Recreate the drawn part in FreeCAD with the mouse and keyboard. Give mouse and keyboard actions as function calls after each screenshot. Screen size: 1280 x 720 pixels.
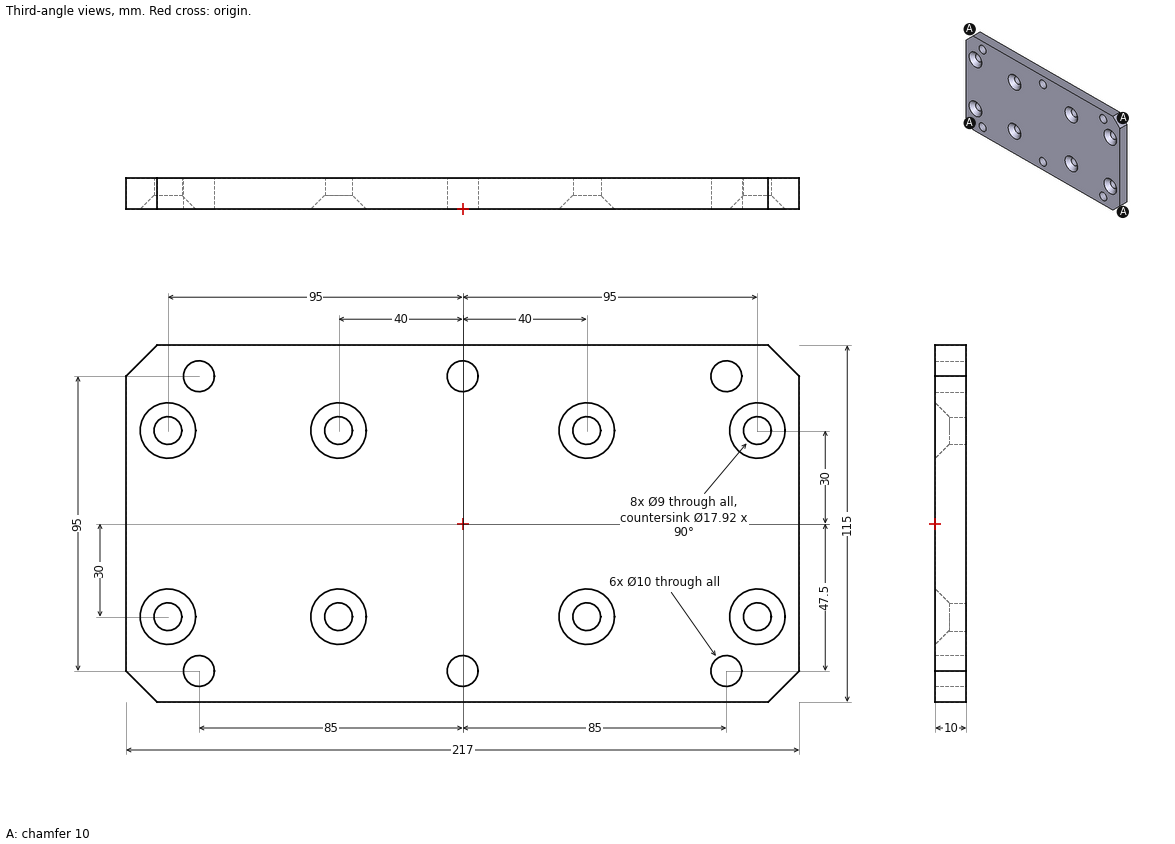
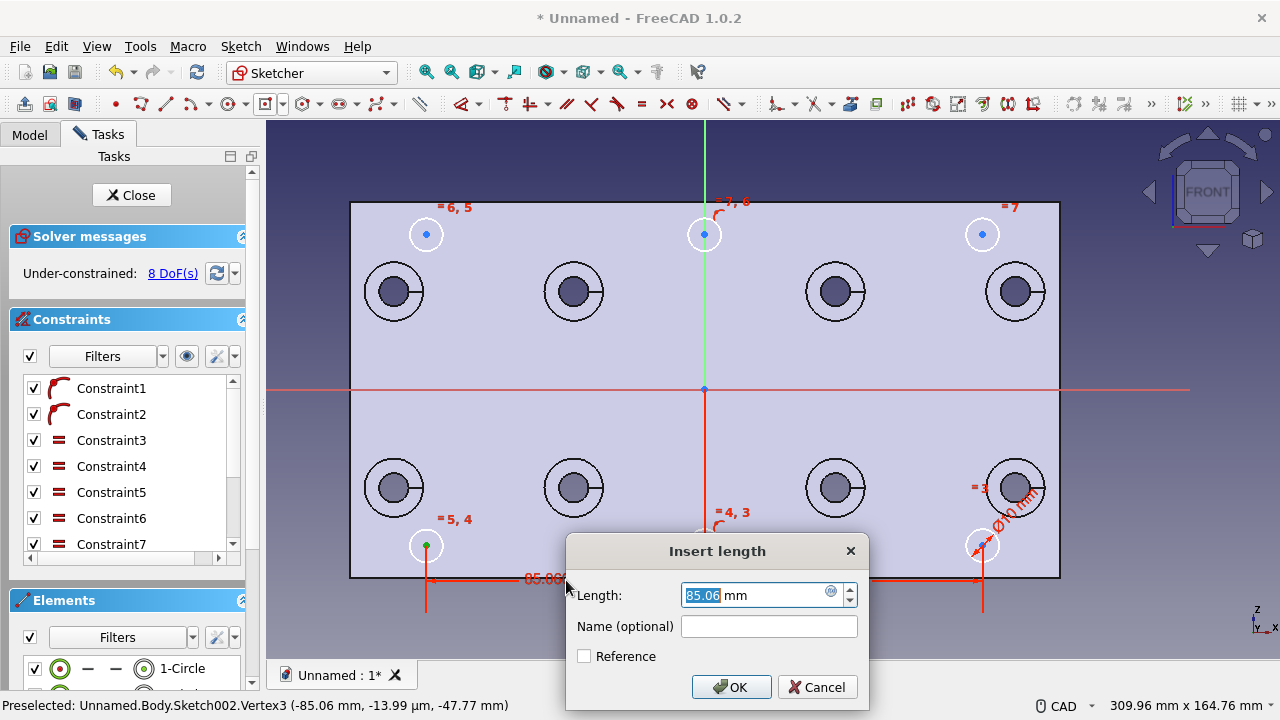
text(85)
key(Return)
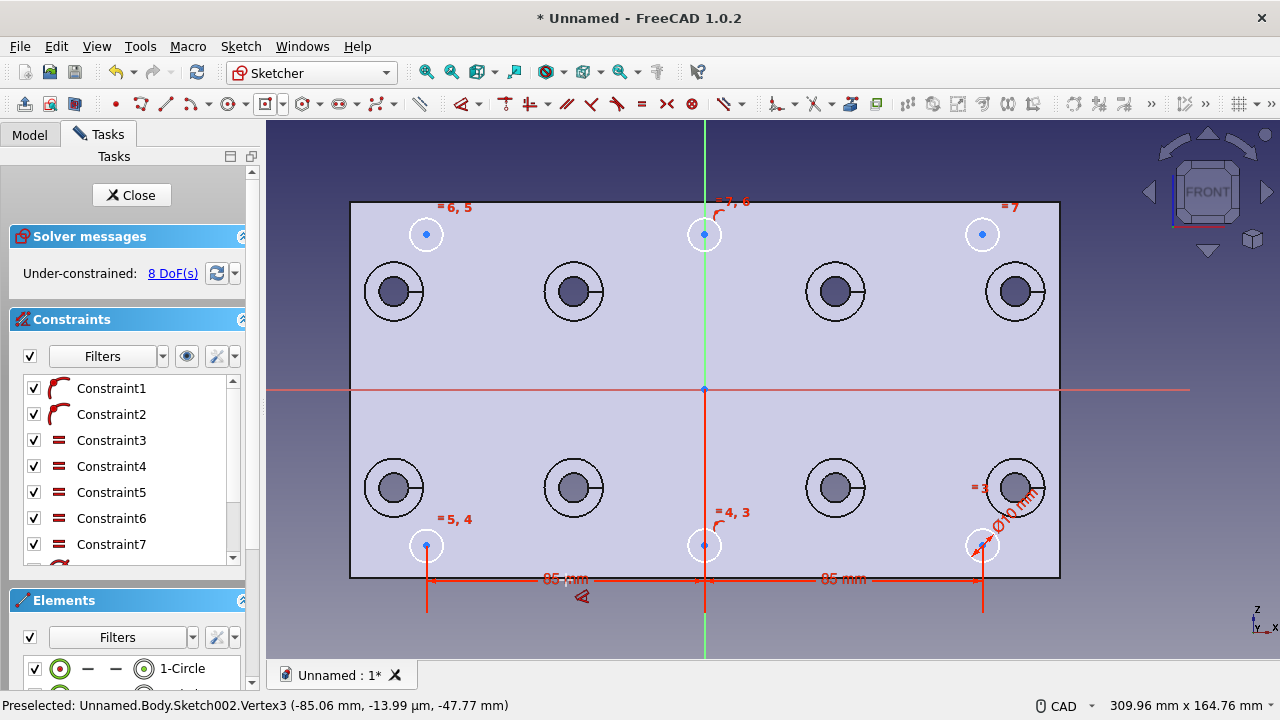
click(426, 235)
click(566, 201)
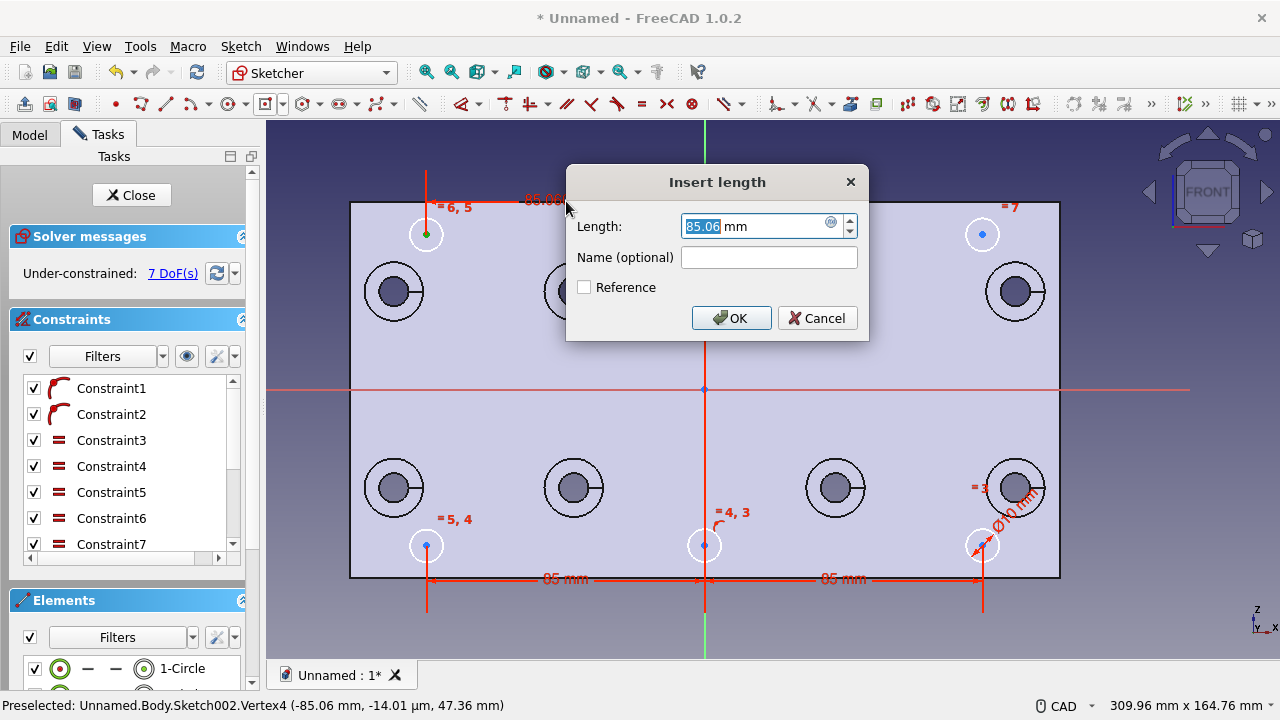
text(85)
key(Return)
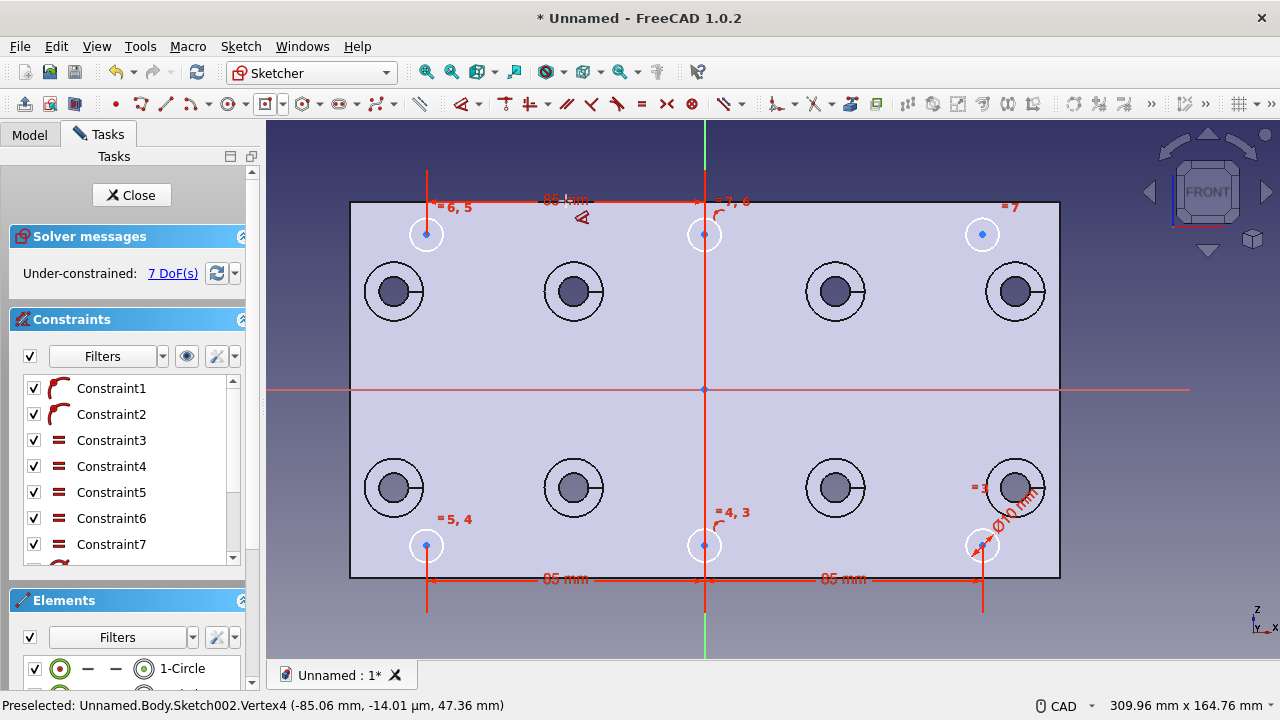
click(983, 235)
click(844, 201)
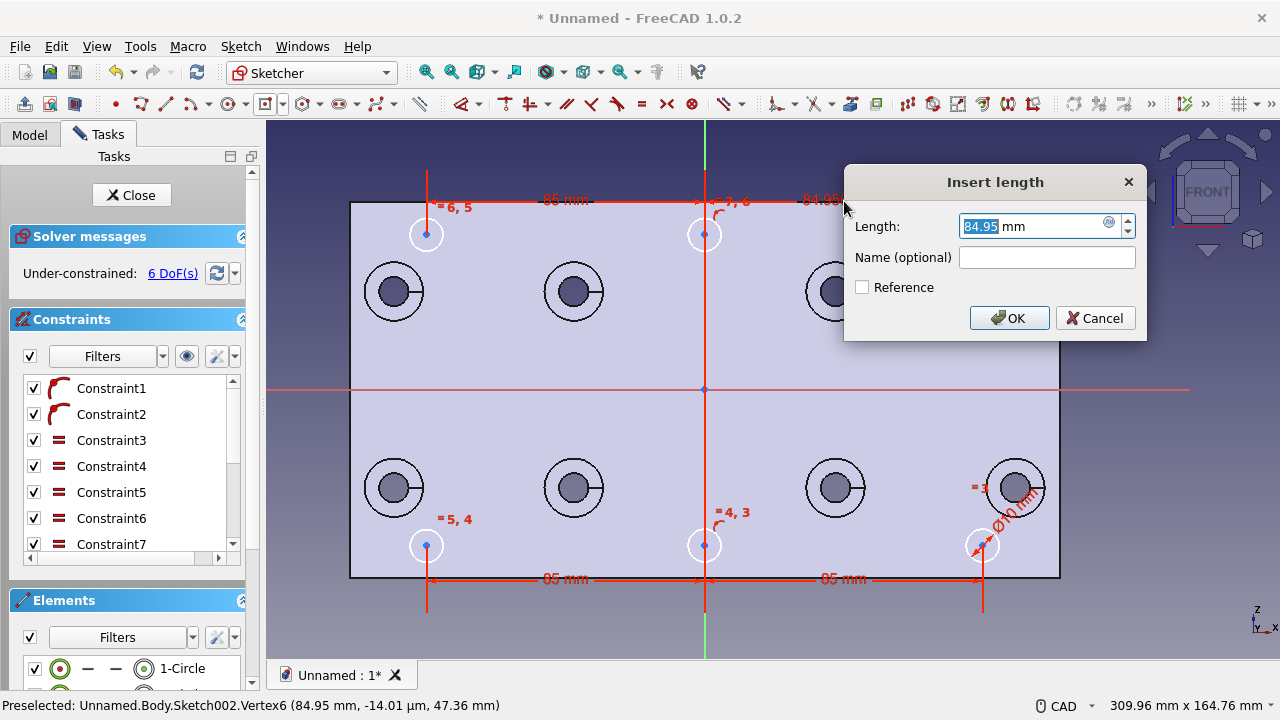
text(85)
key(Return)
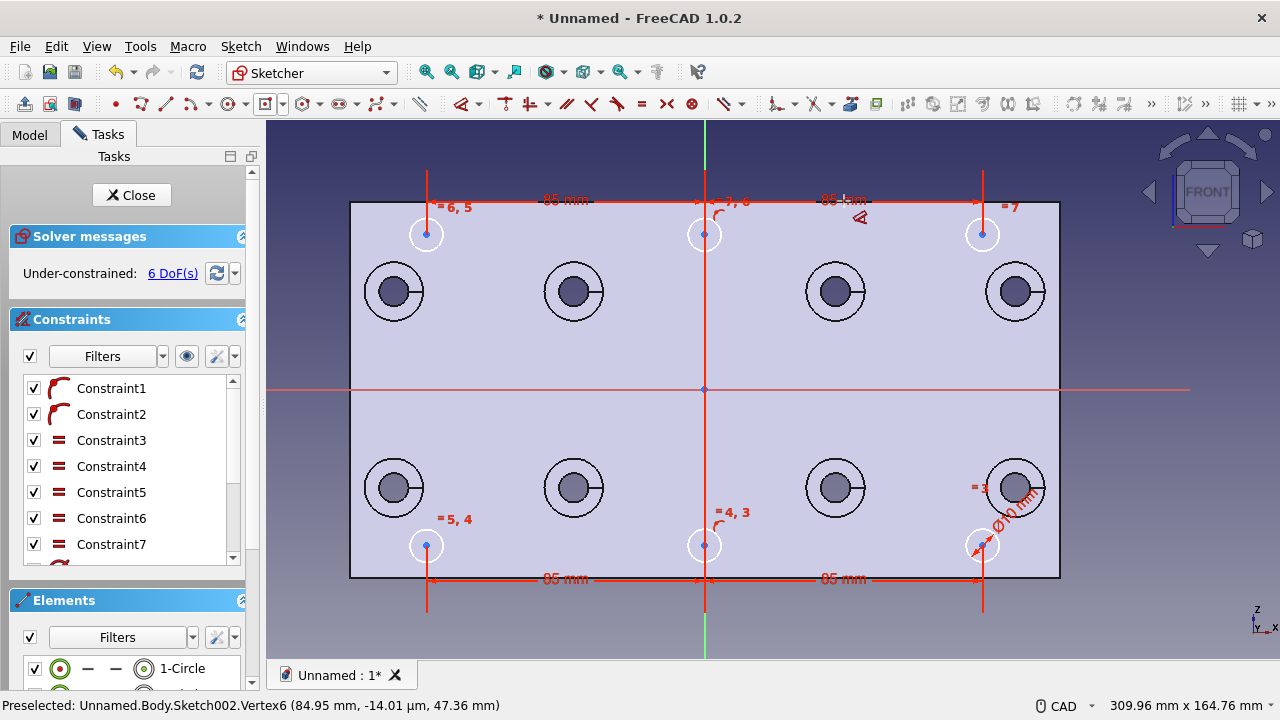
click(427, 546)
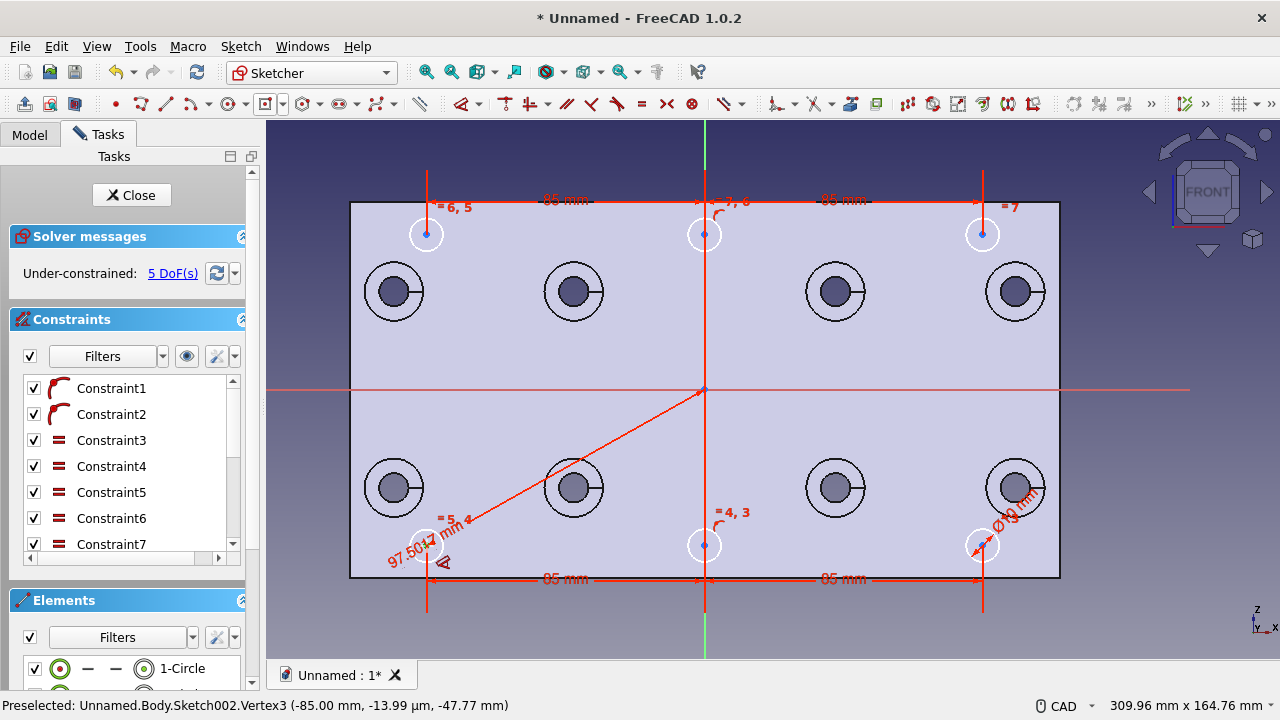
click(427, 235)
click(393, 319)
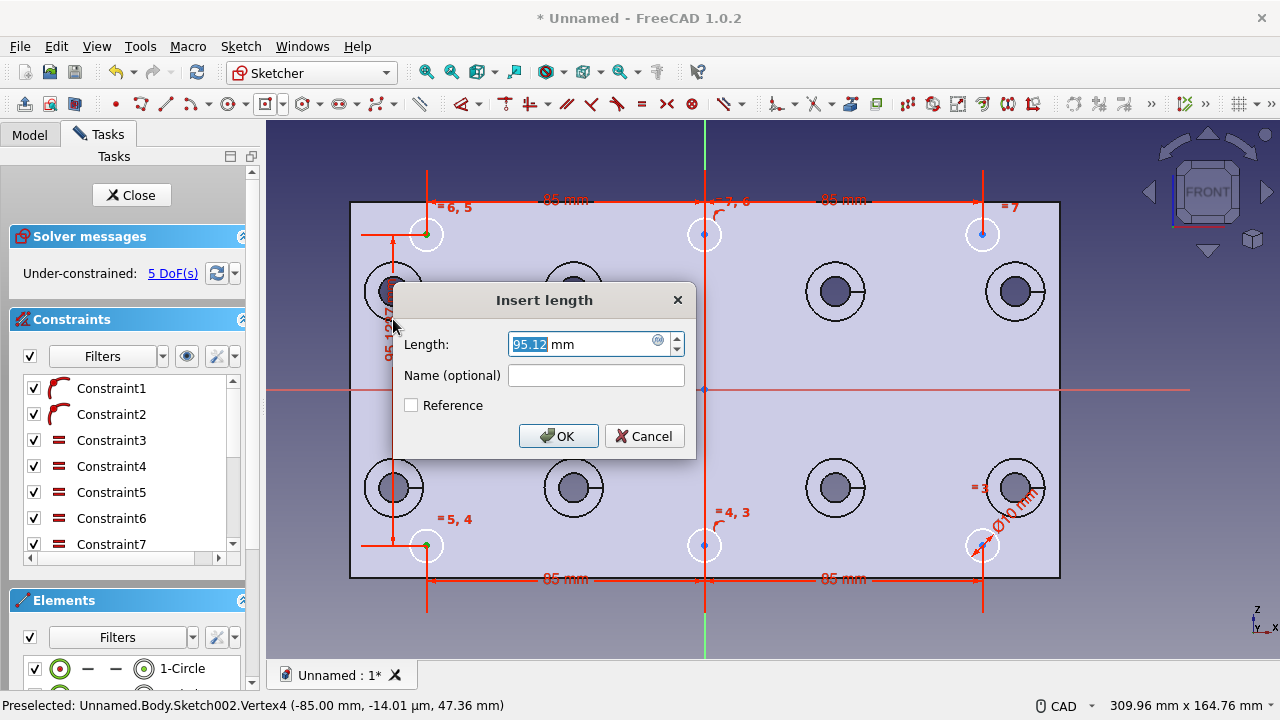
text(95)
key(Return)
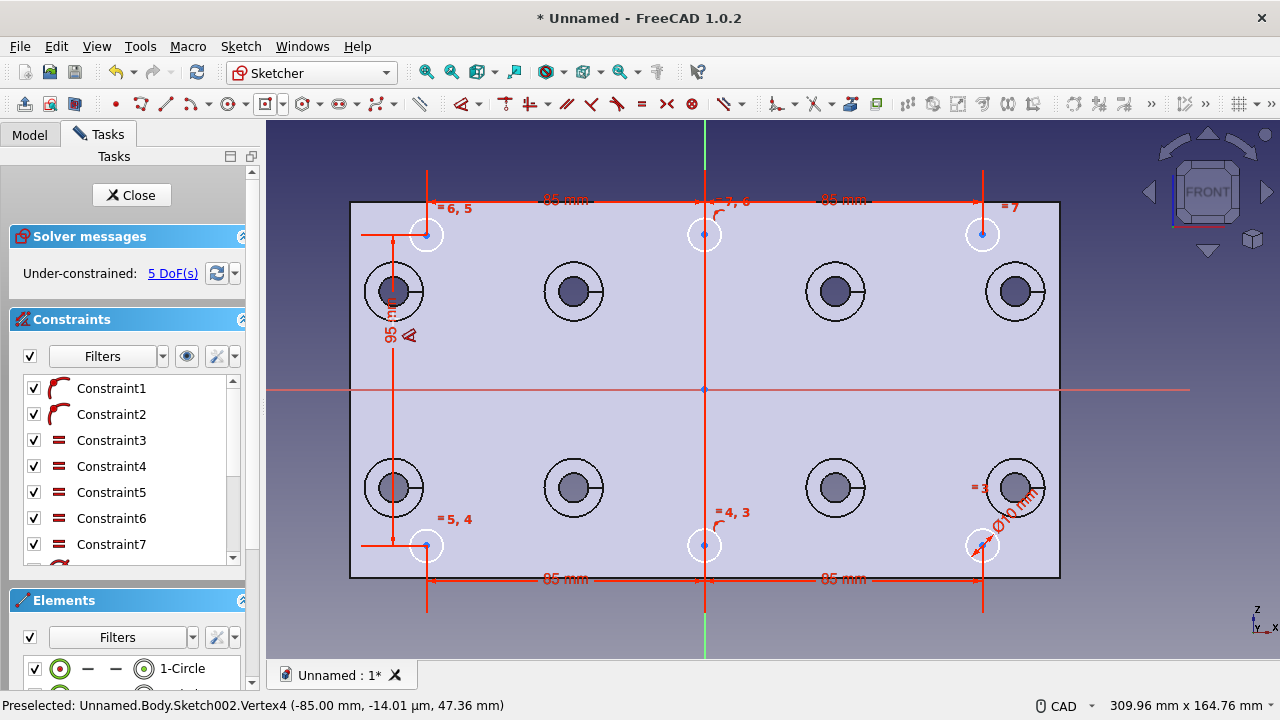
click(705, 546)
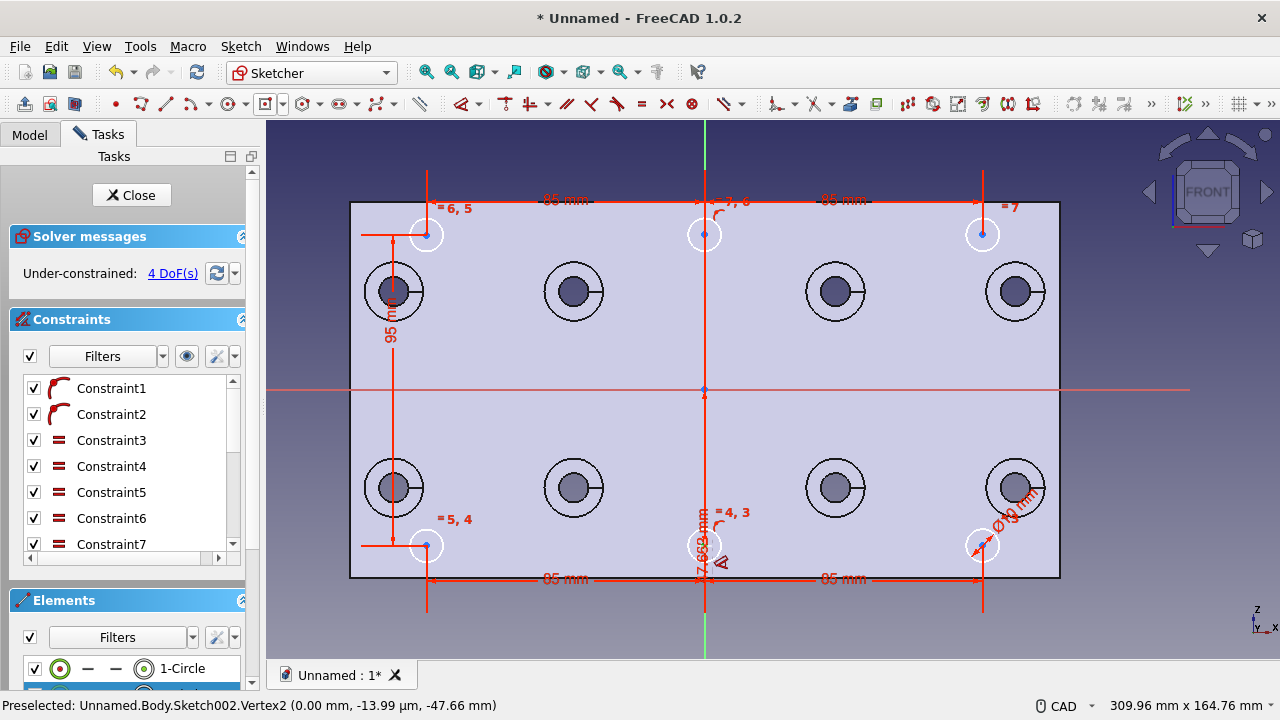
click(427, 235)
click(393, 462)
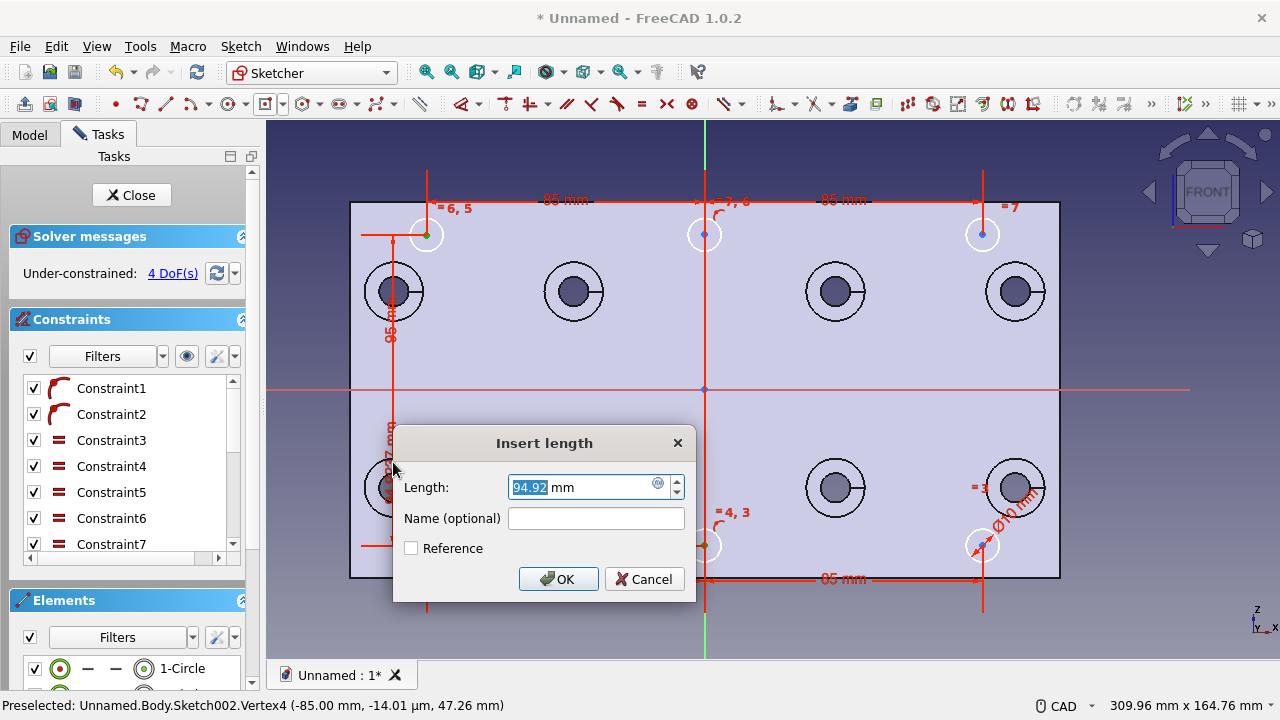
text(95)
key(Return)